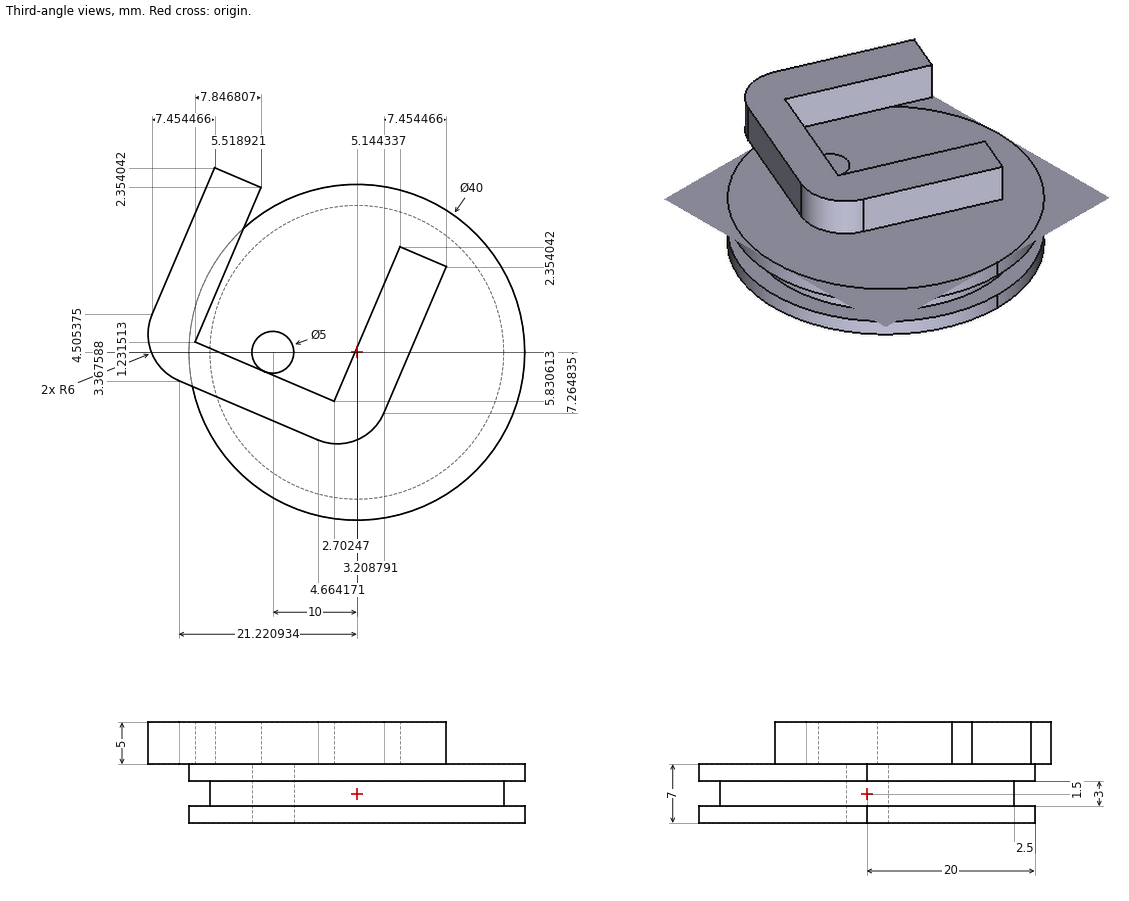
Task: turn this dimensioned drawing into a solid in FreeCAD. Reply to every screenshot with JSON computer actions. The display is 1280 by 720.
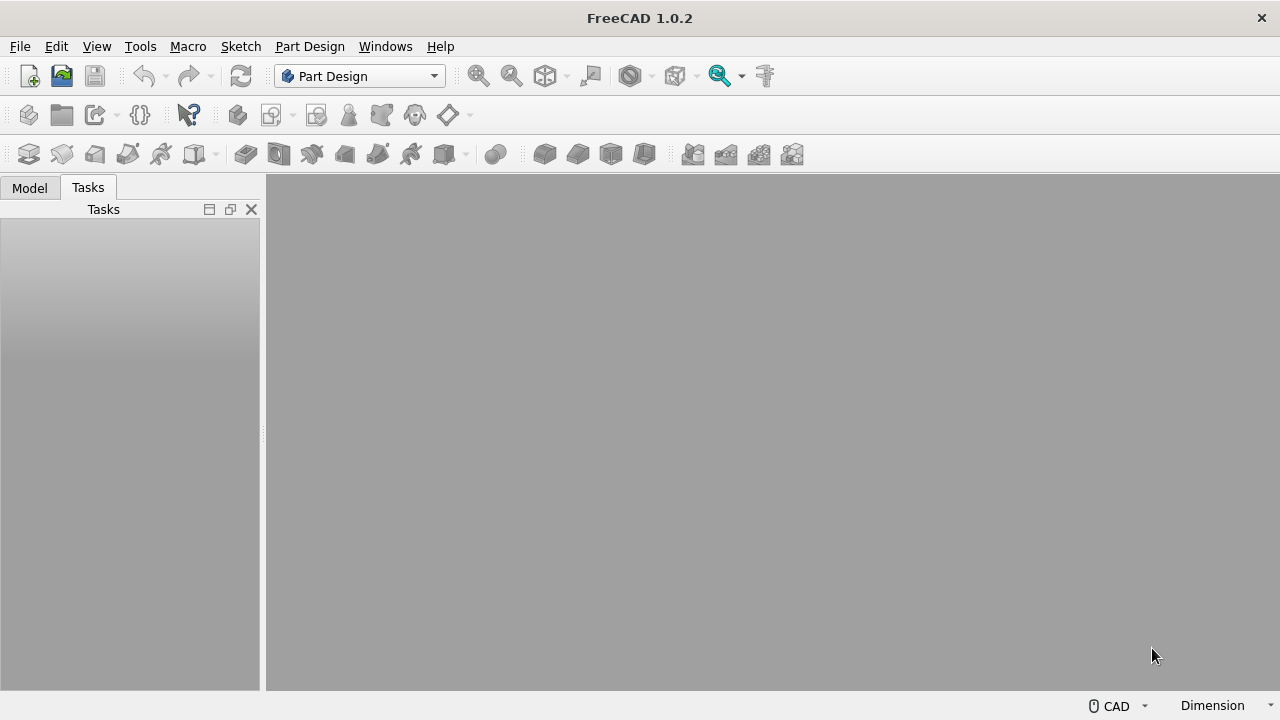
{"action": "left_click", "coordinate": [29, 76]}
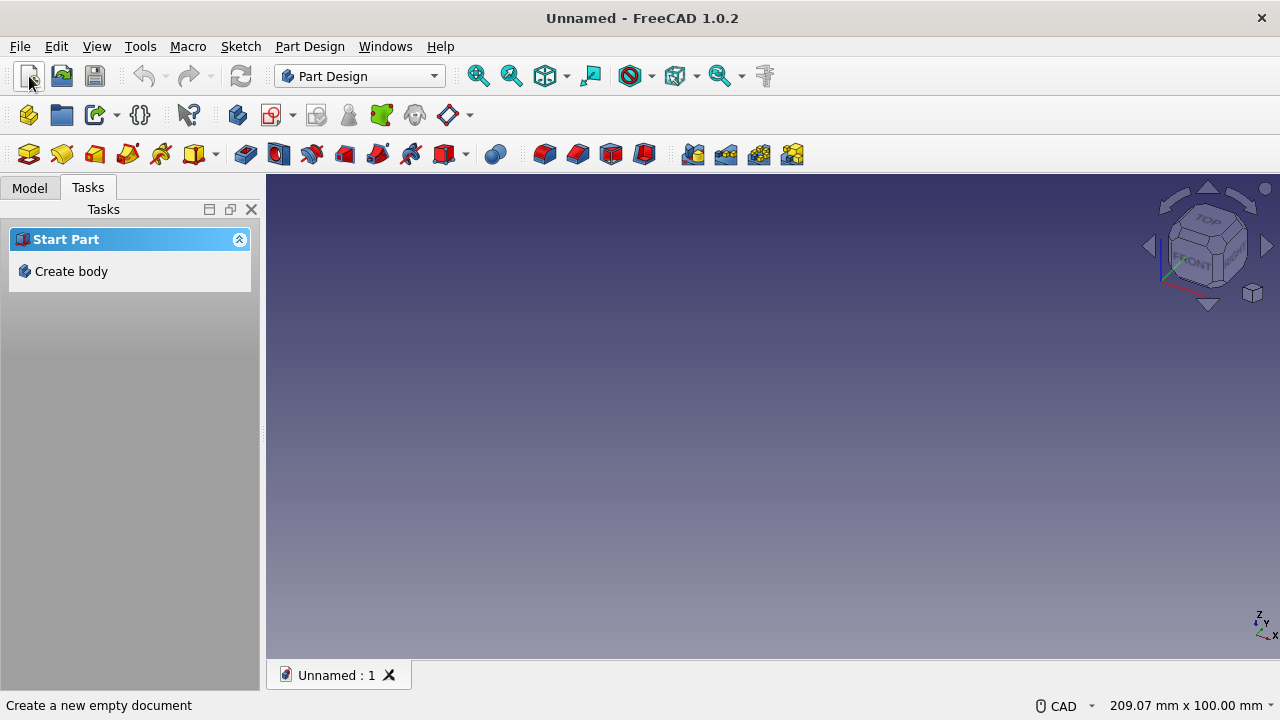
{"action": "left_click", "coordinate": [270, 116]}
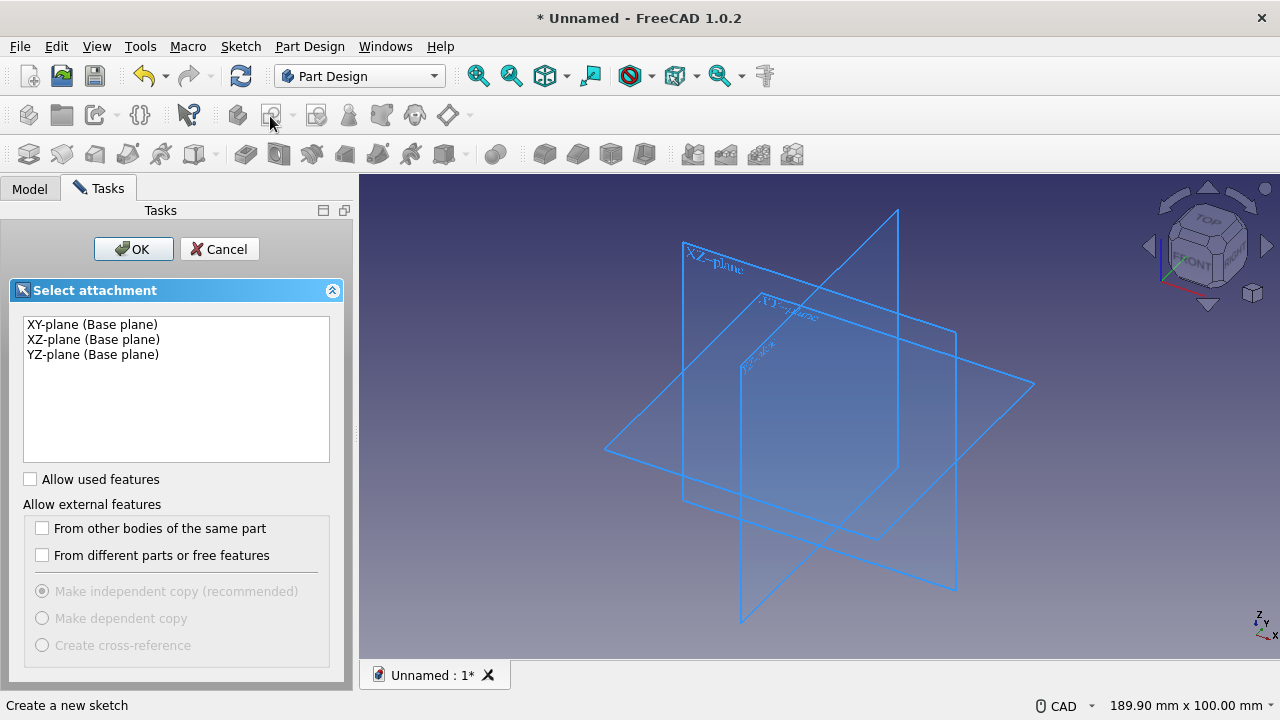
{"action": "left_click", "coordinate": [84, 324]}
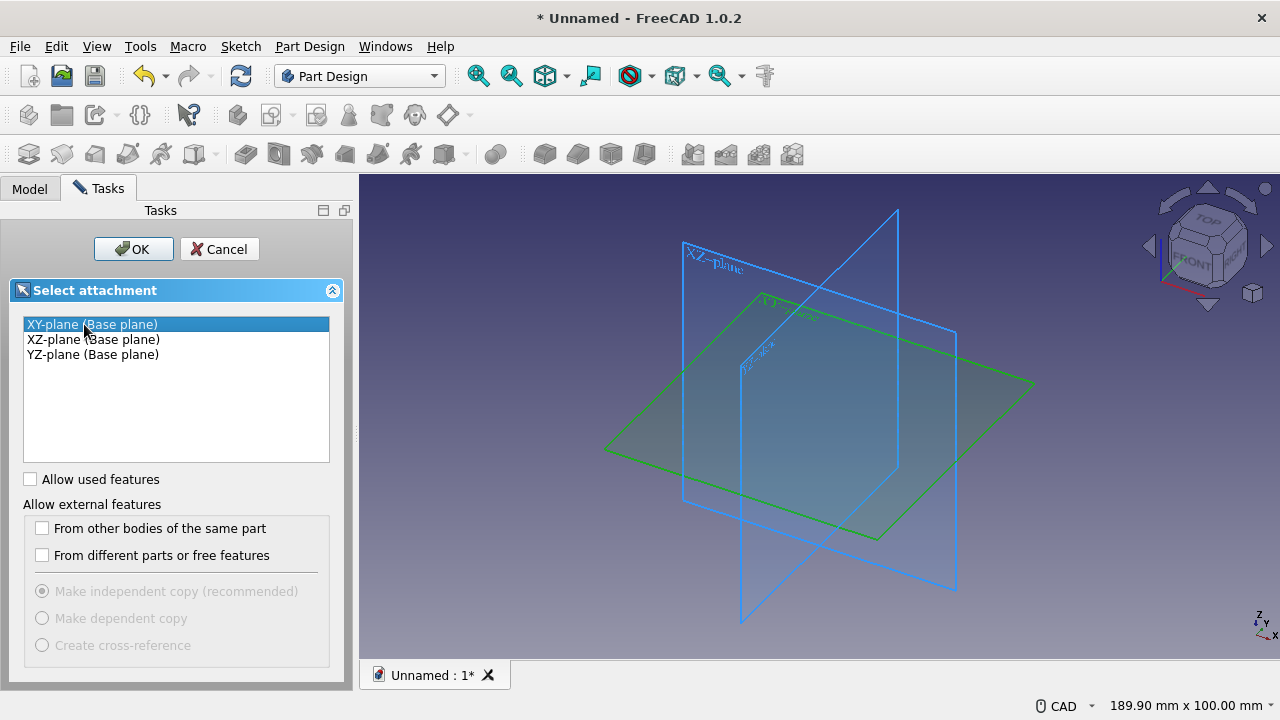
{"action": "left_click", "coordinate": [134, 249]}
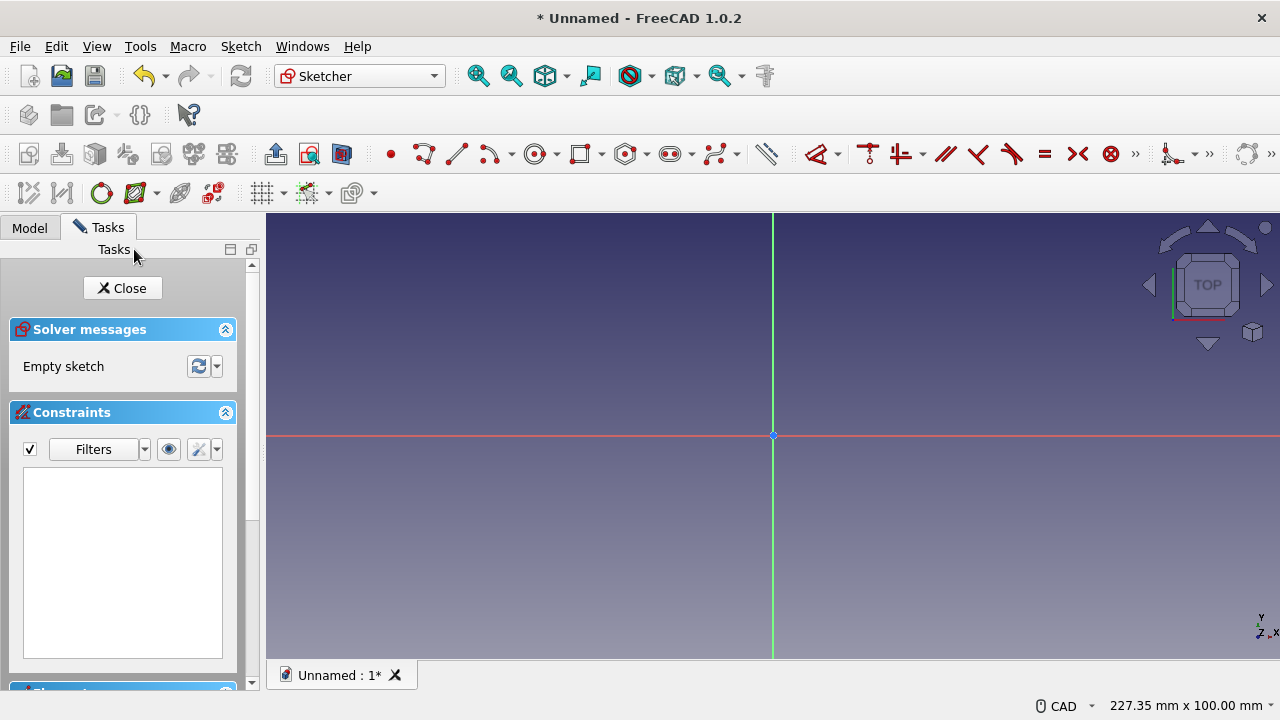
{"action": "scroll", "coordinate": [912, 436], "scroll_direction": "up", "scroll_amount": 2}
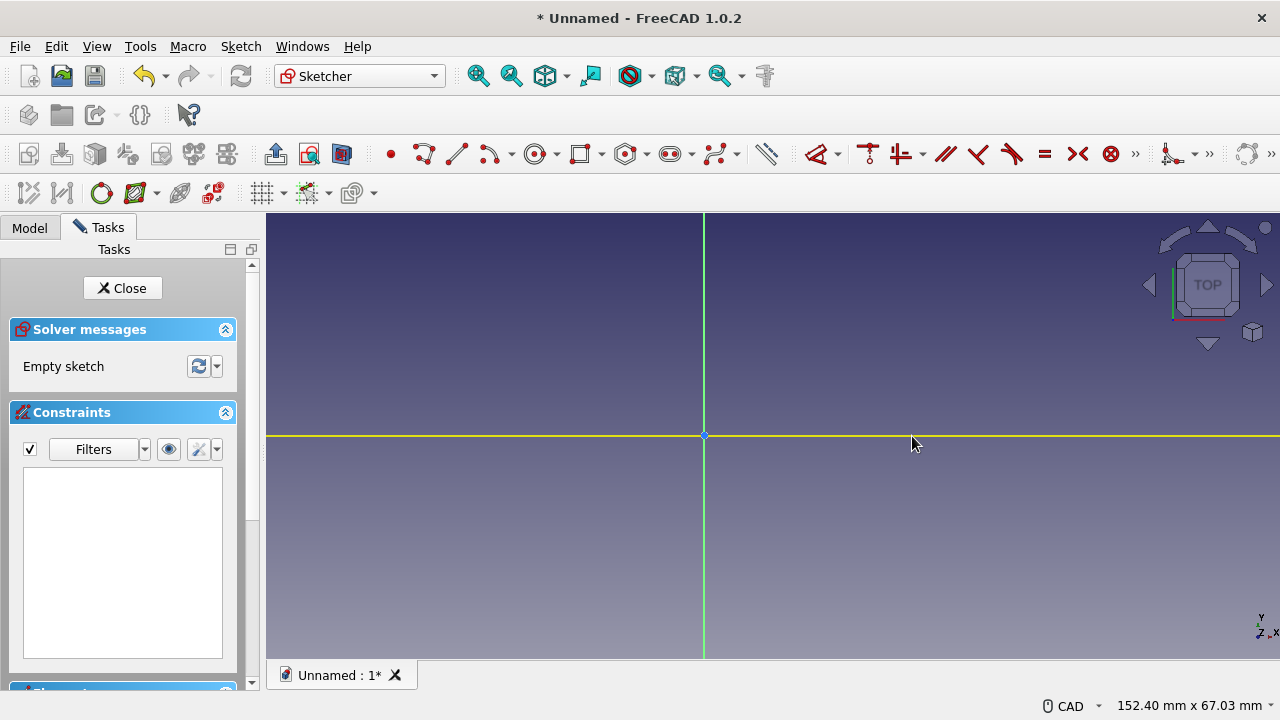
{"action": "left_click", "coordinate": [534, 154]}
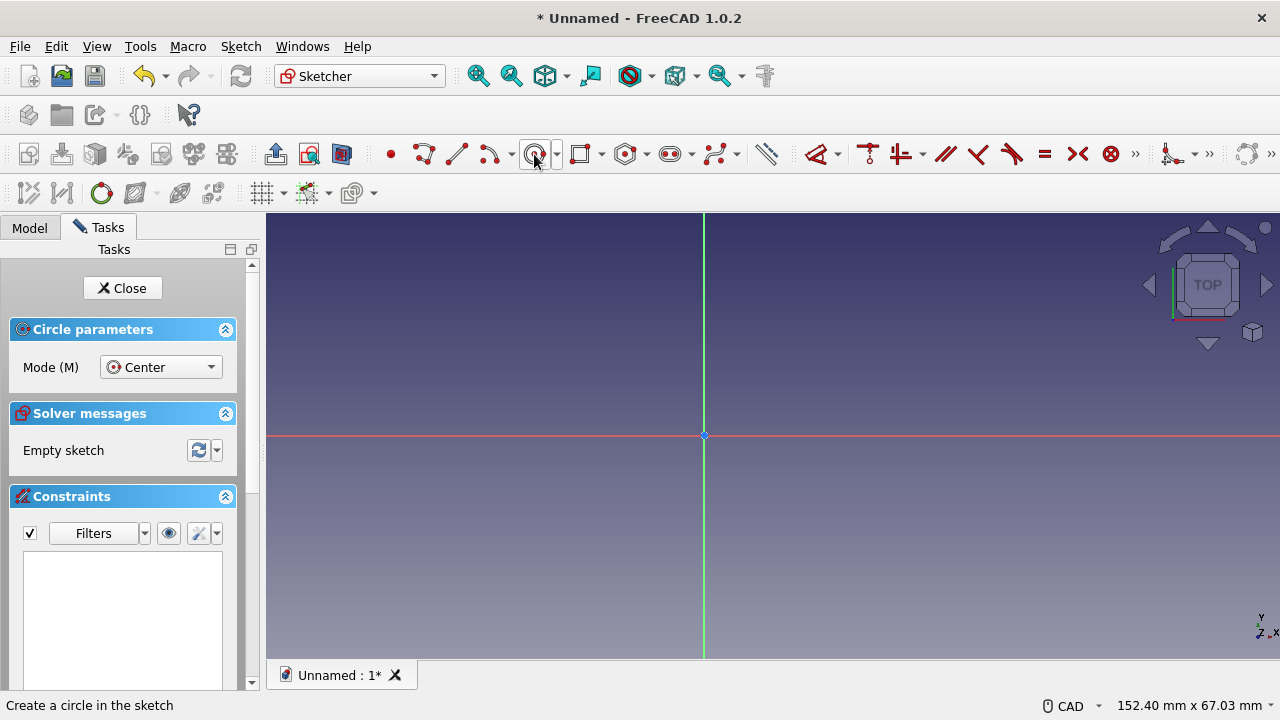
{"action": "left_click", "coordinate": [704, 436]}
{"action": "left_click", "coordinate": [798, 342]}
{"action": "key", "text": "Escape"}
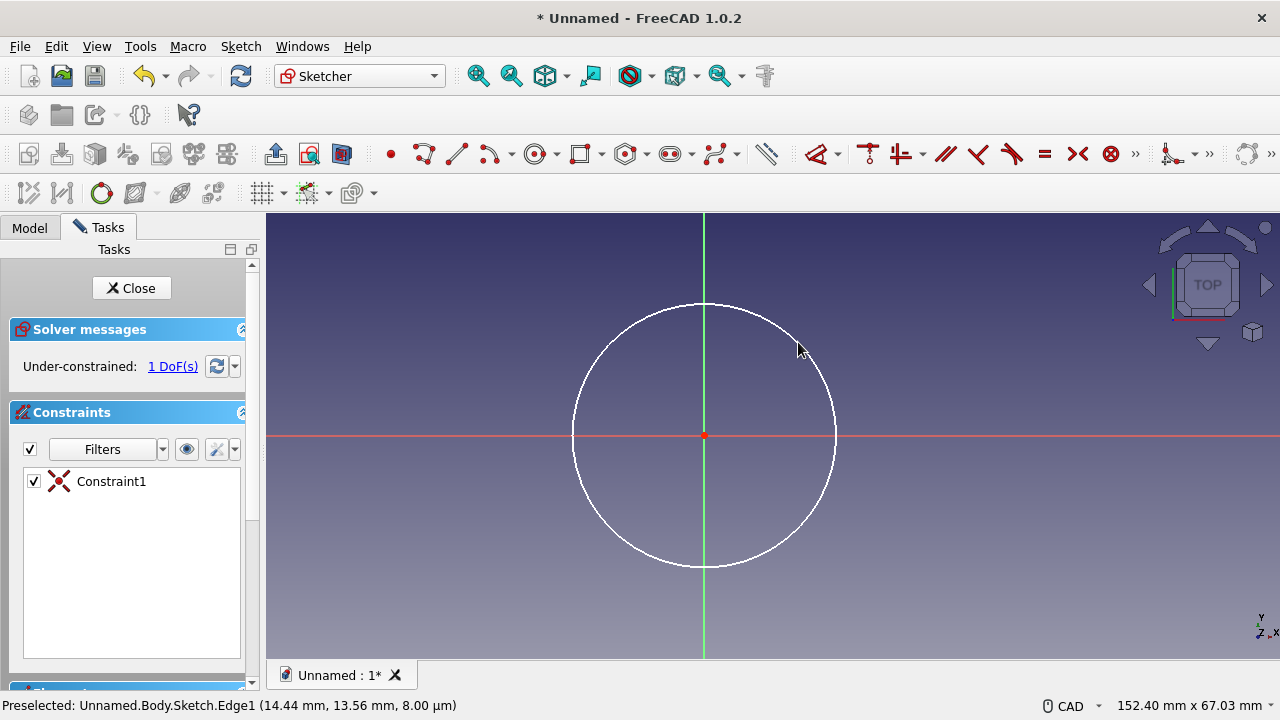
{"action": "left_click", "coordinate": [816, 154]}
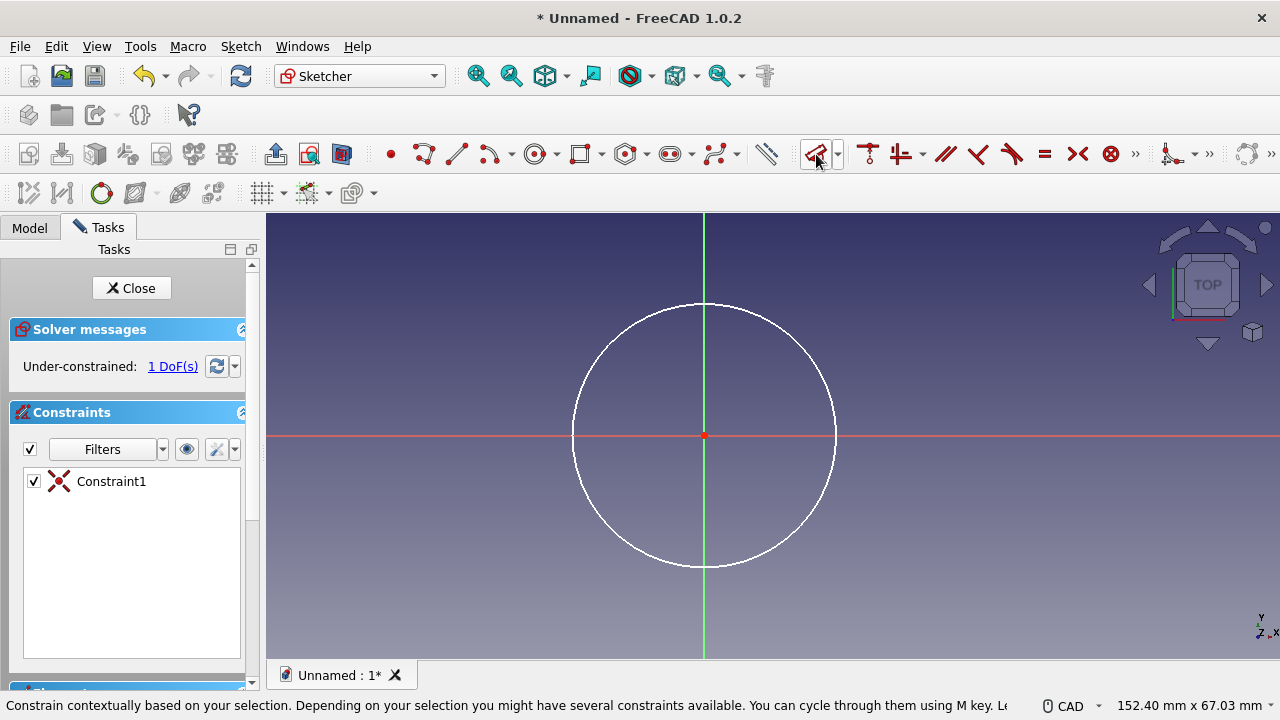
{"action": "left_click", "coordinate": [797, 342]}
{"action": "left_click", "coordinate": [819, 319]}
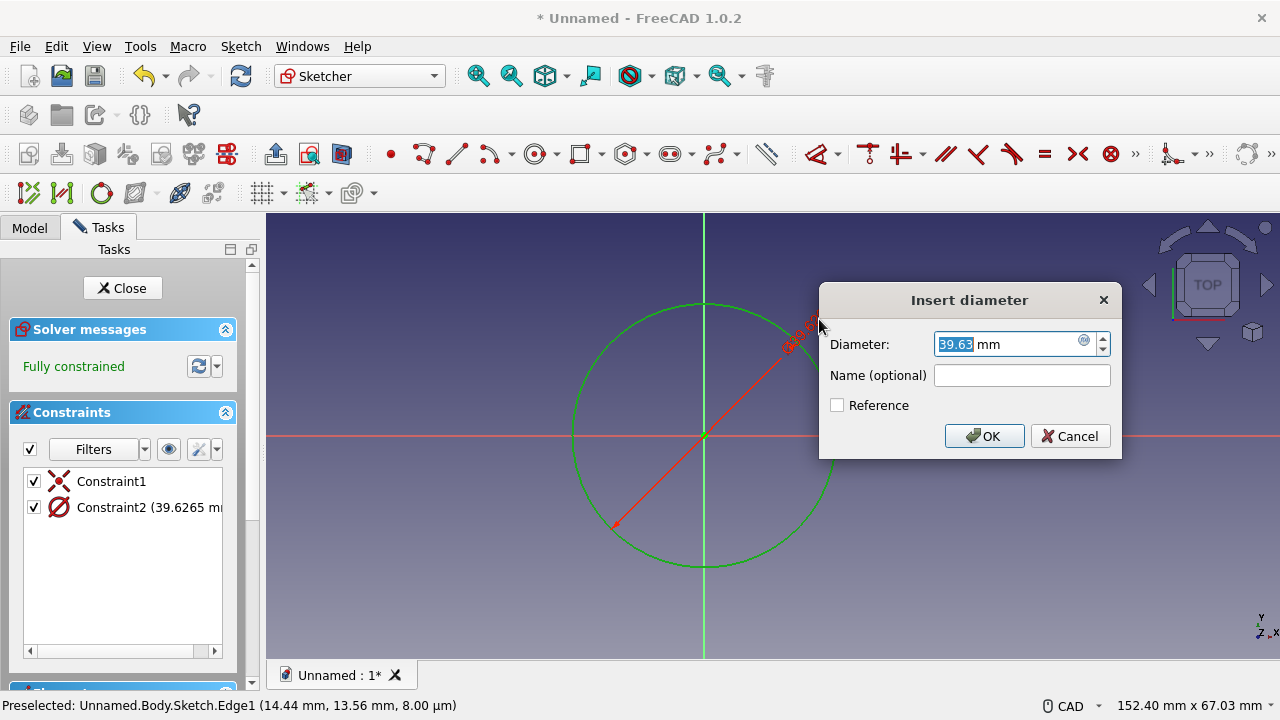
{"action": "type", "text": "40"}
{"action": "key", "text": "Return"}
{"action": "key", "text": "Escape"}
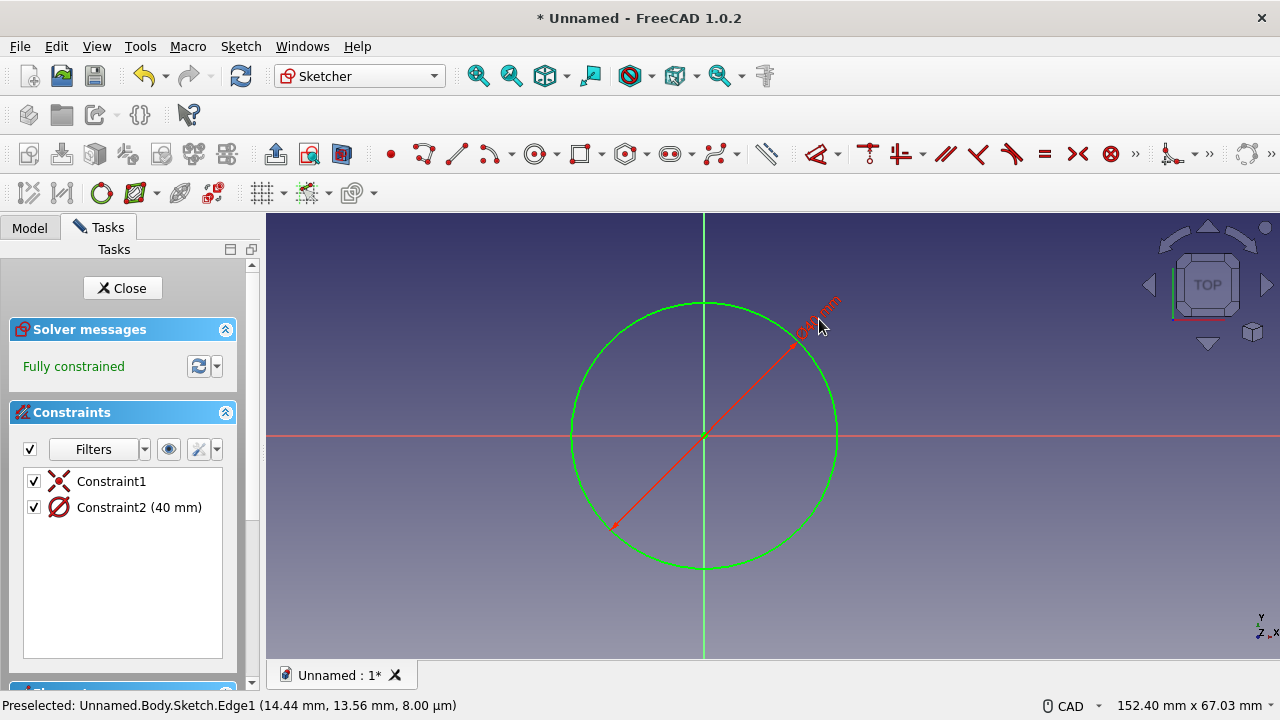
{"action": "left_click", "coordinate": [123, 288]}